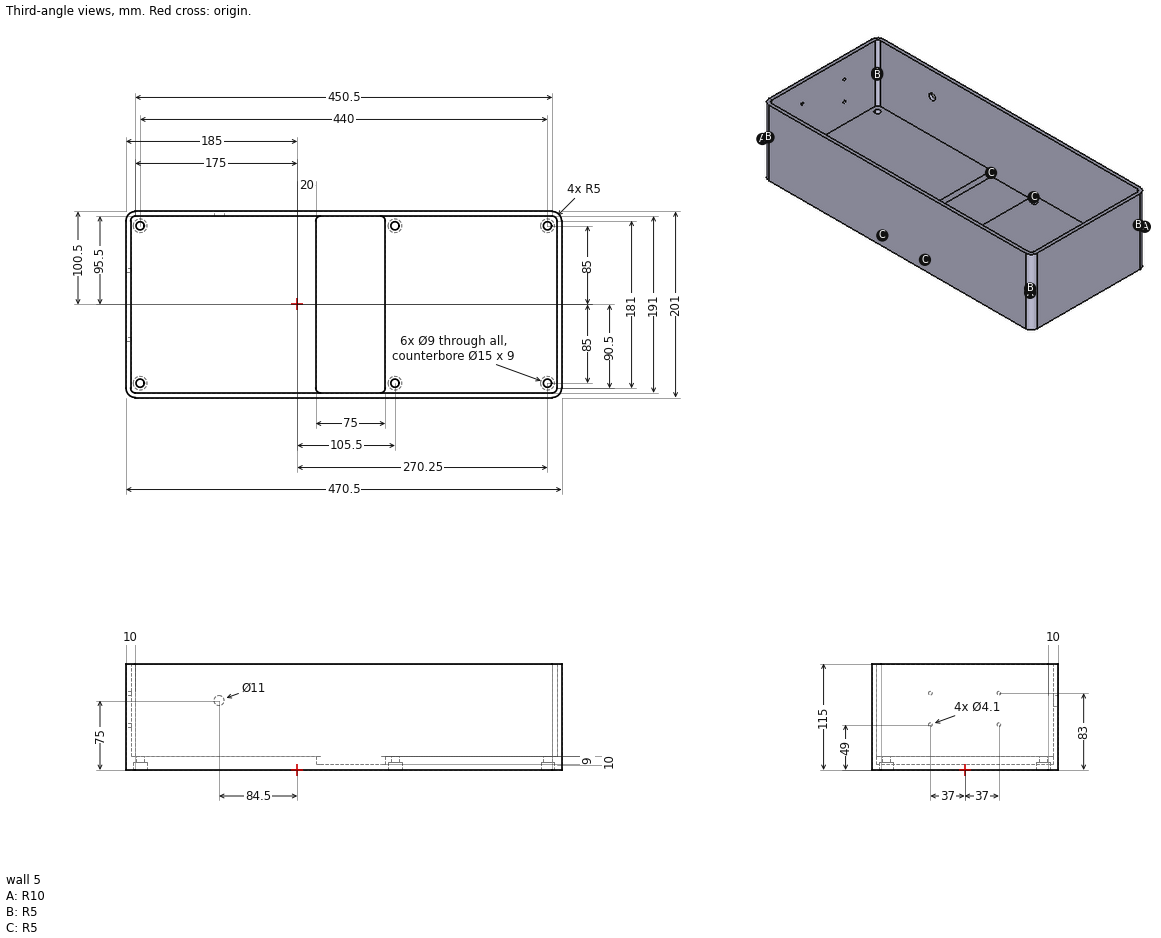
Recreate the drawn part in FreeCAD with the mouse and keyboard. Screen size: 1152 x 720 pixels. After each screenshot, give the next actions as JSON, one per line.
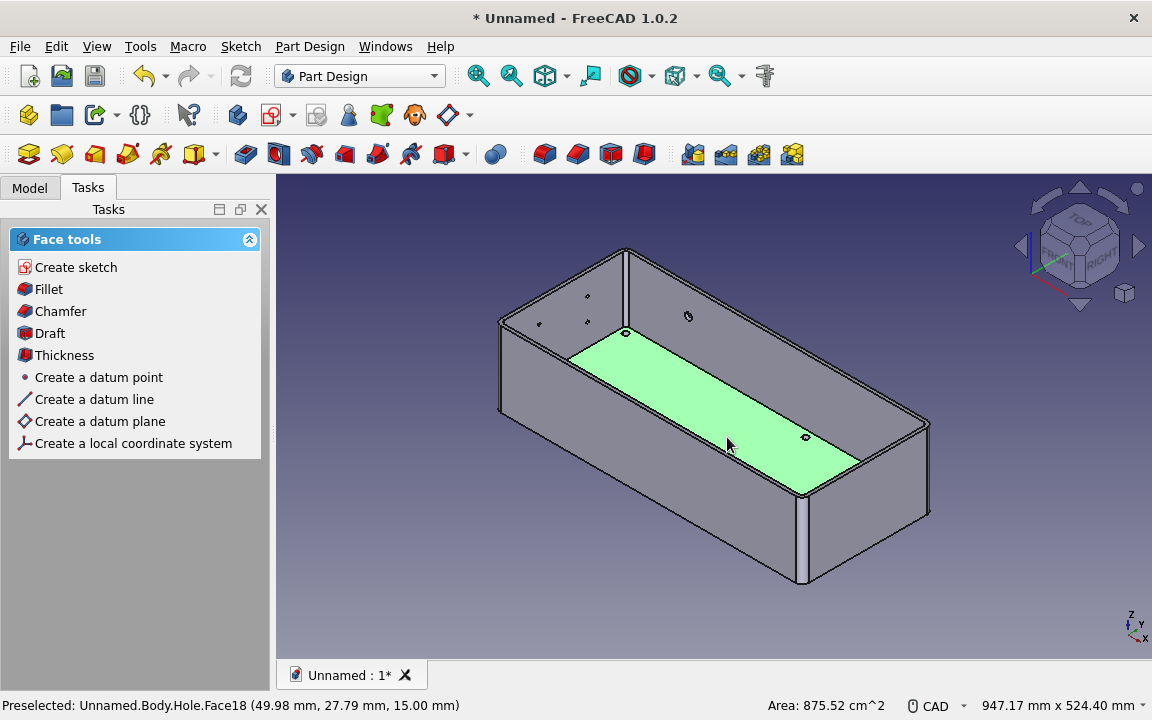
{"action": "left_click", "coordinate": [270, 116]}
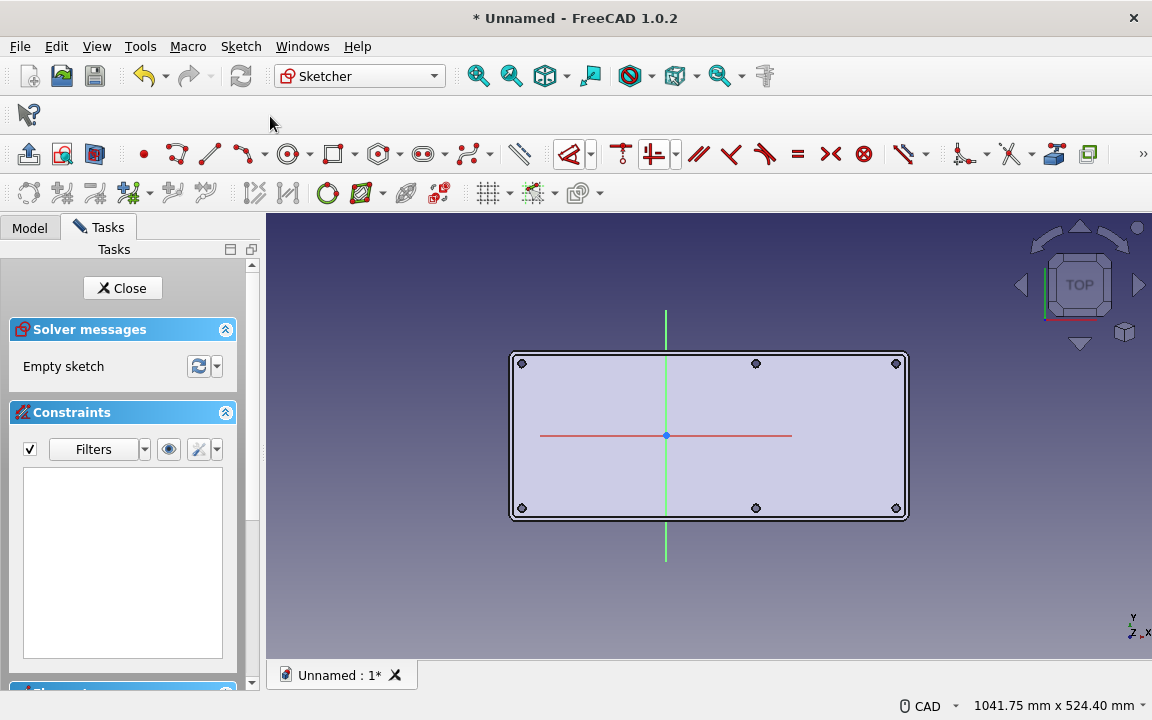
{"action": "scroll", "coordinate": [787, 436], "scroll_direction": "up", "scroll_amount": 3}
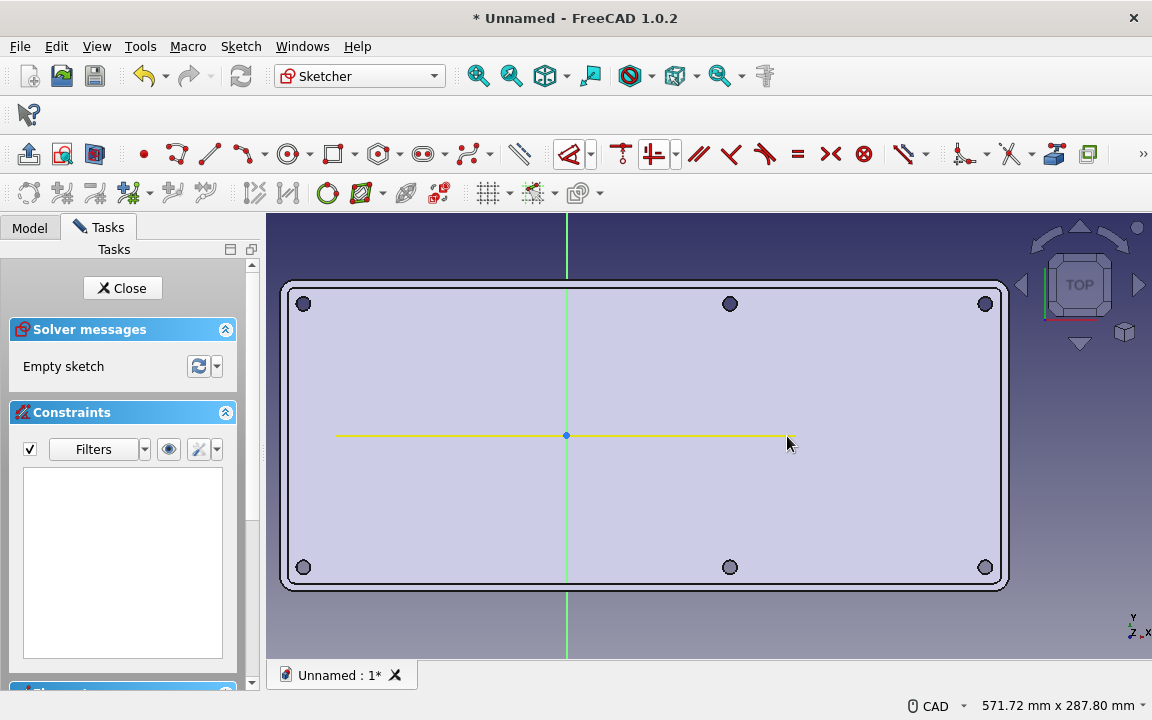
{"action": "left_click", "coordinate": [332, 154]}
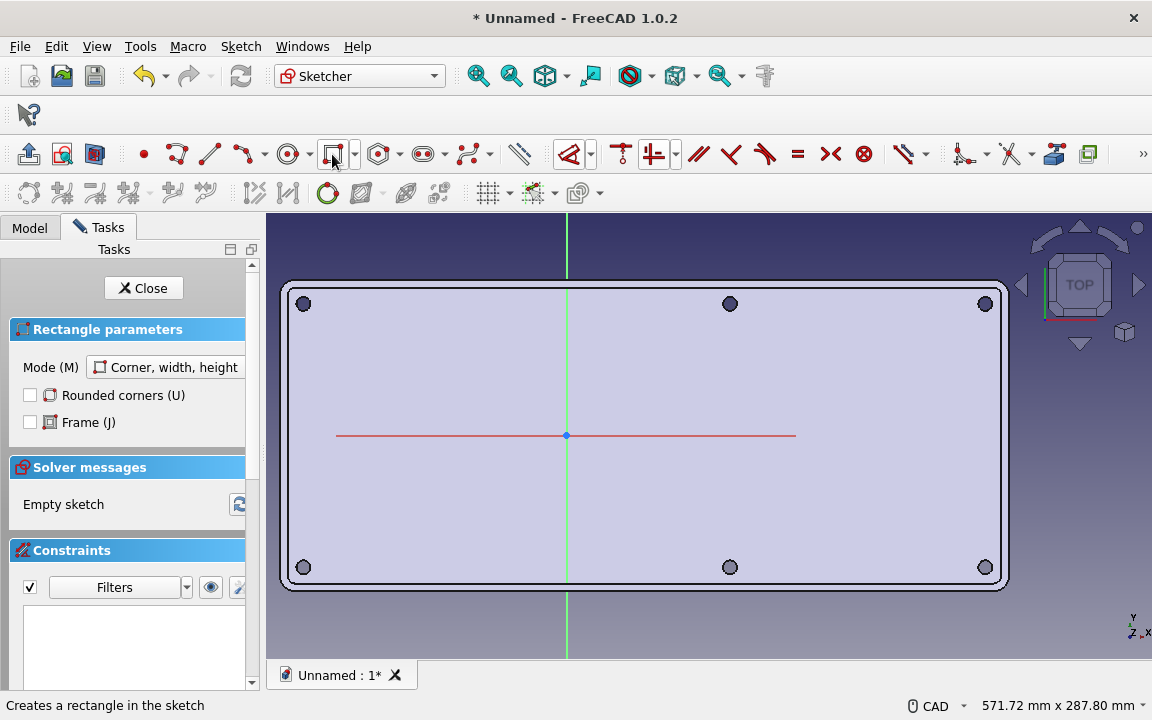
{"action": "left_click", "coordinate": [598, 288]}
{"action": "mouse_move", "coordinate": [714, 584]}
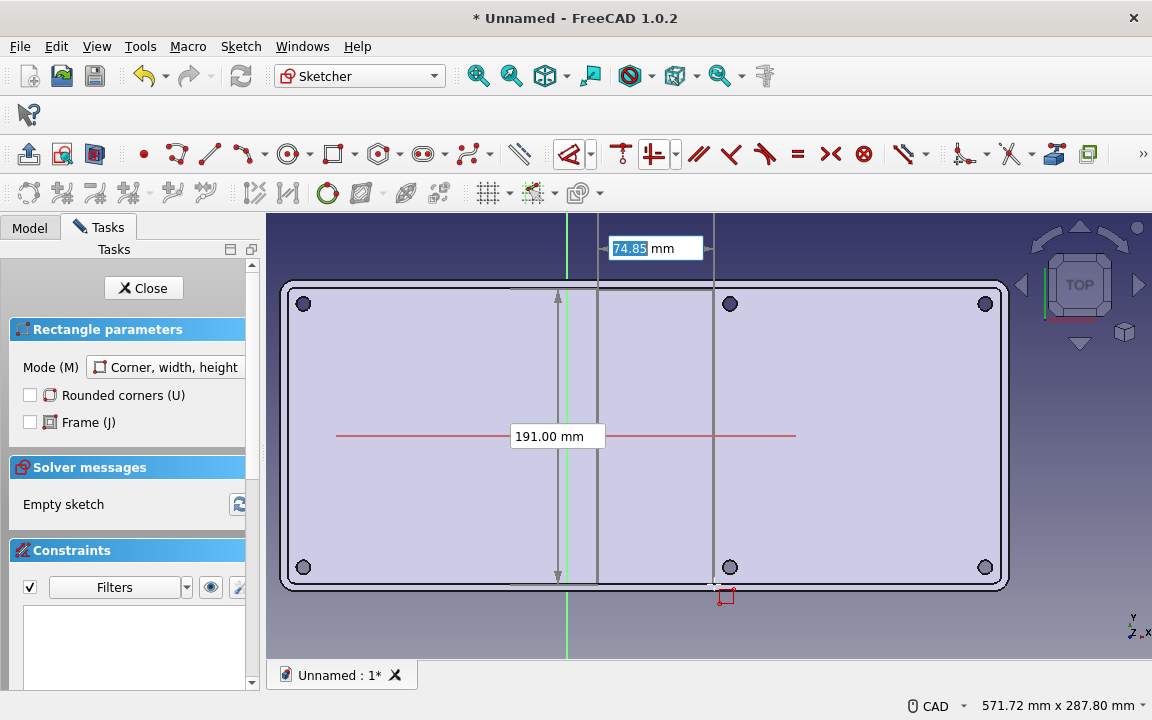
{"action": "type", "text": "75"}
{"action": "key", "text": "Tab"}
{"action": "type", "text": "191"}
{"action": "key", "text": "Return"}
{"action": "key", "text": "Escape"}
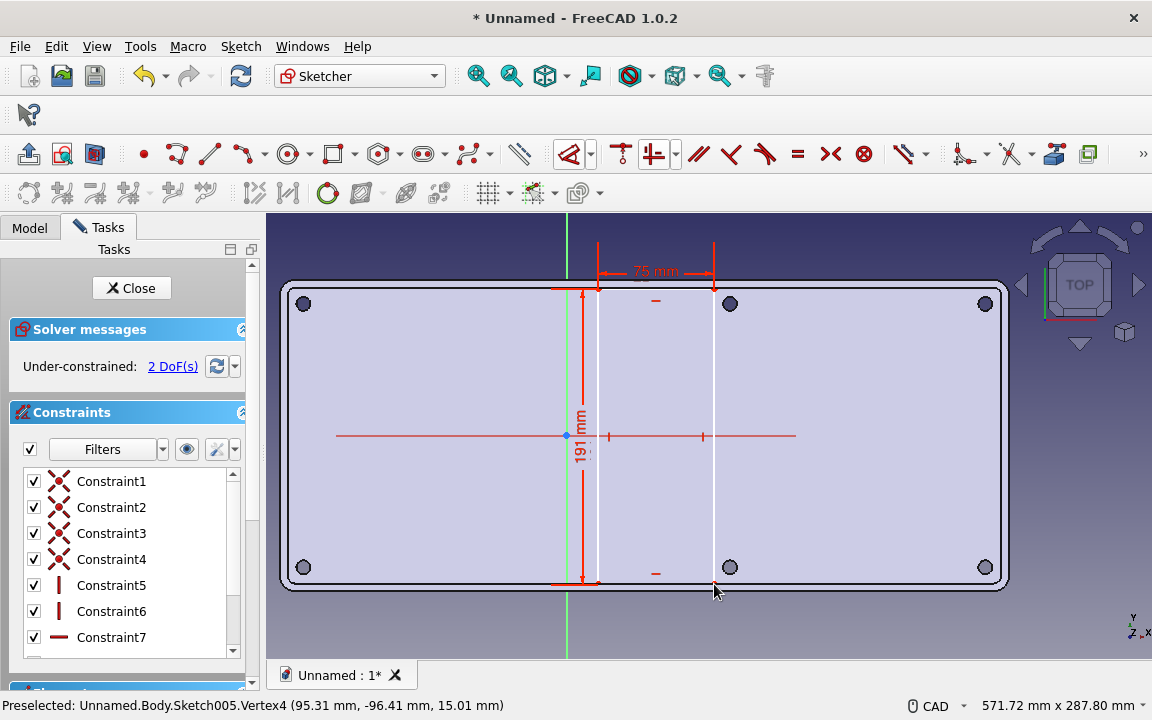
{"action": "key", "text": "d"}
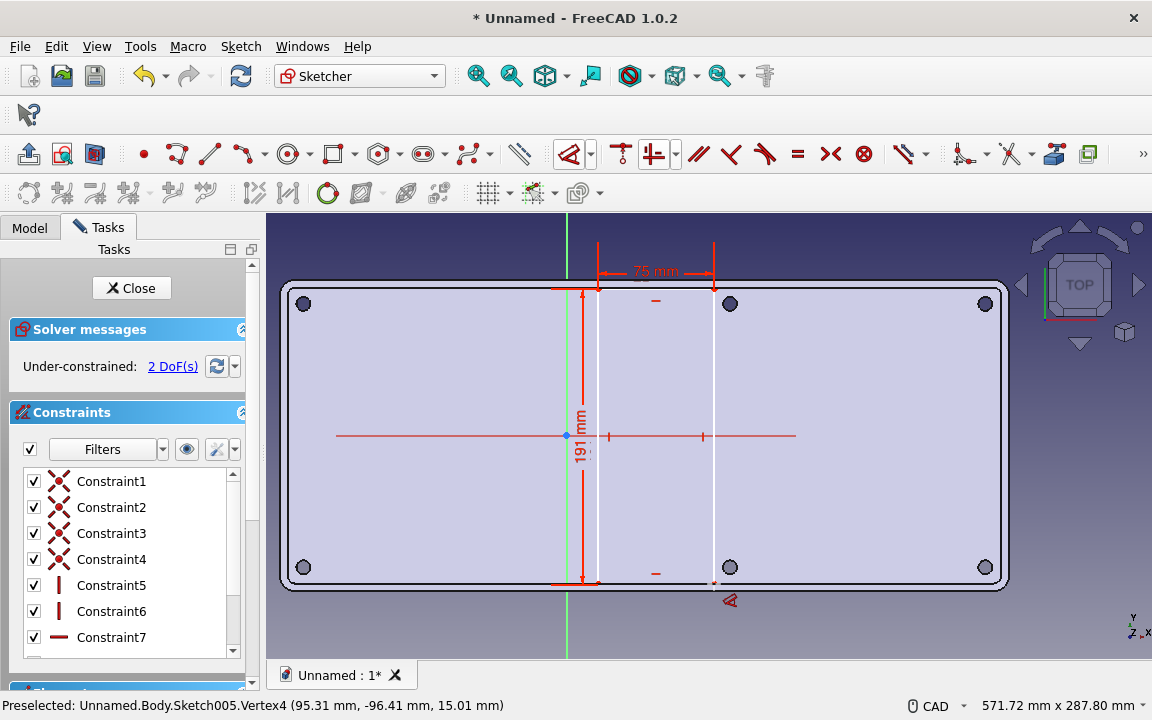
{"action": "scroll", "coordinate": [598, 289], "scroll_direction": "up", "scroll_amount": 2}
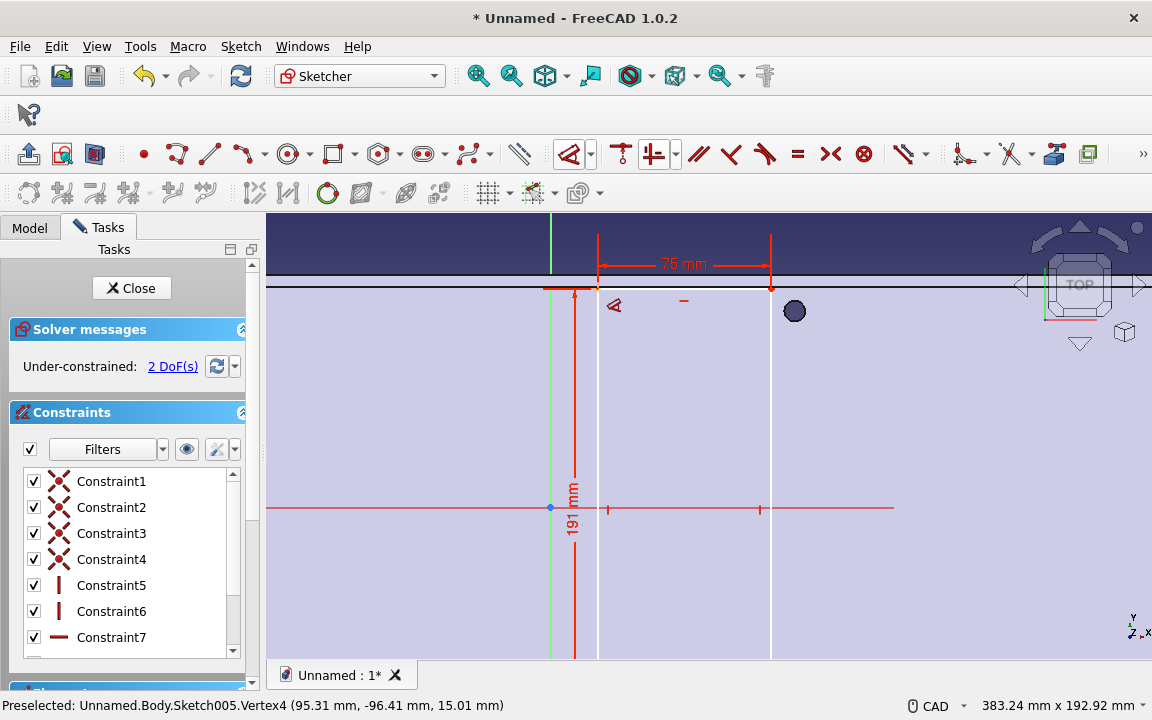
{"action": "left_click", "coordinate": [598, 289]}
{"action": "left_click", "coordinate": [574, 255]}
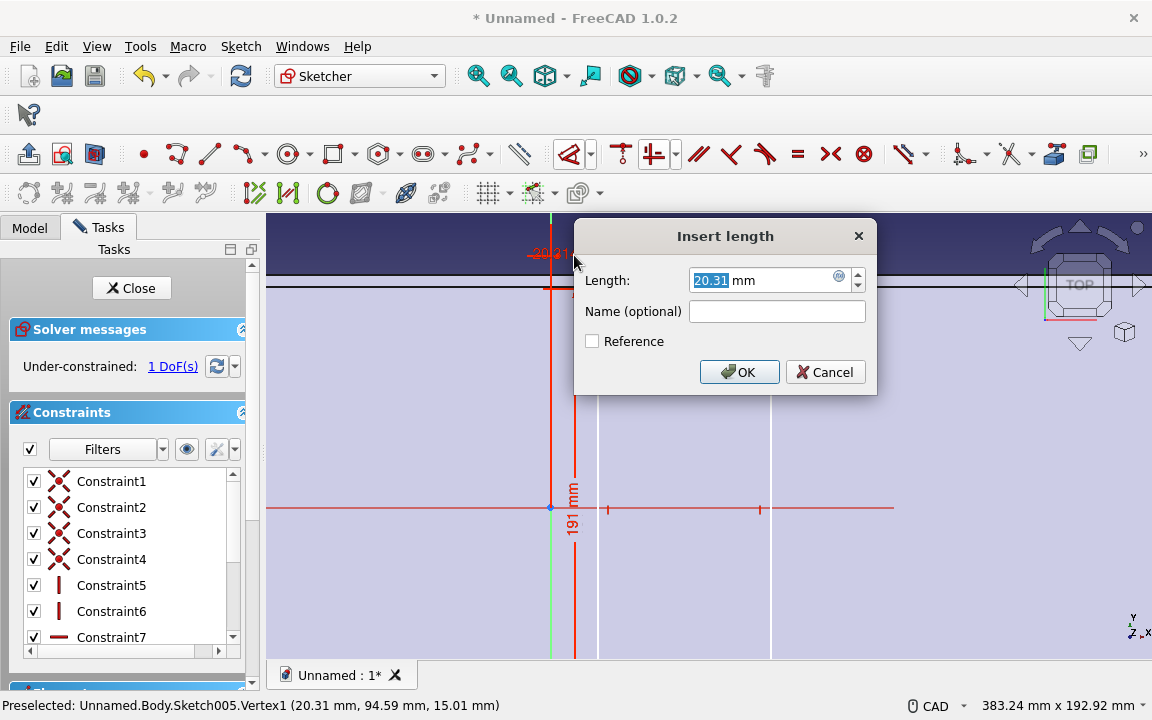
{"action": "type", "text": "20"}
{"action": "key", "text": "Return"}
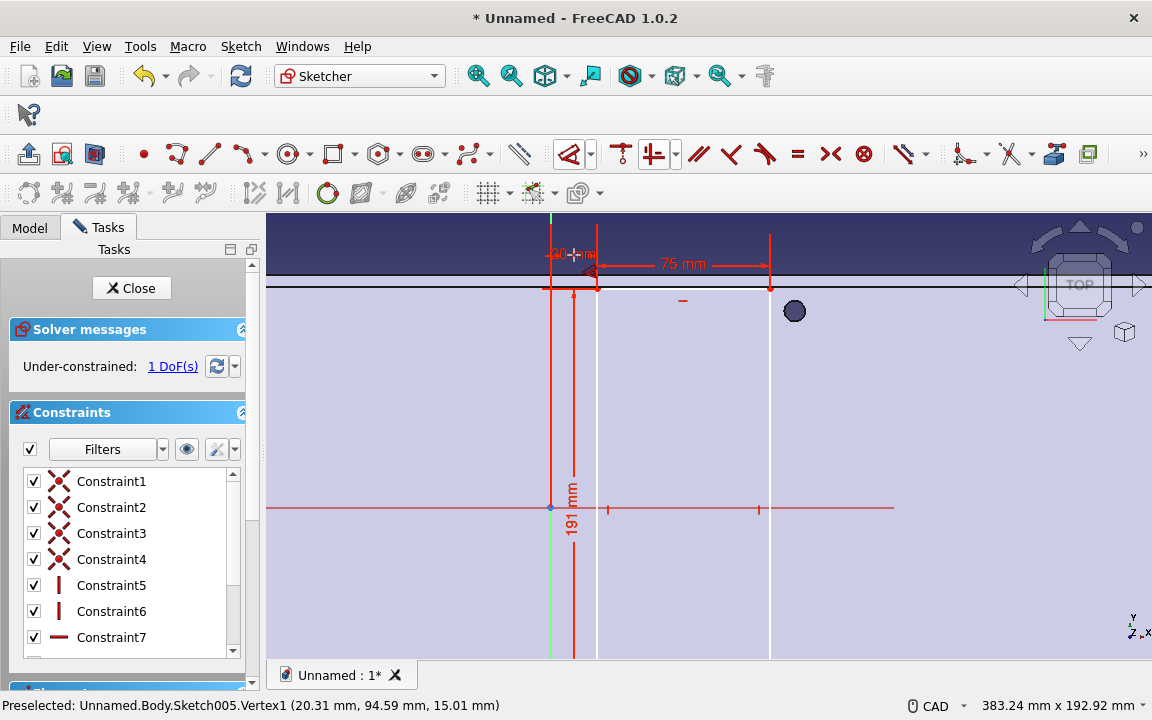
{"action": "left_click", "coordinate": [597, 289]}
{"action": "left_click", "coordinate": [517, 398]}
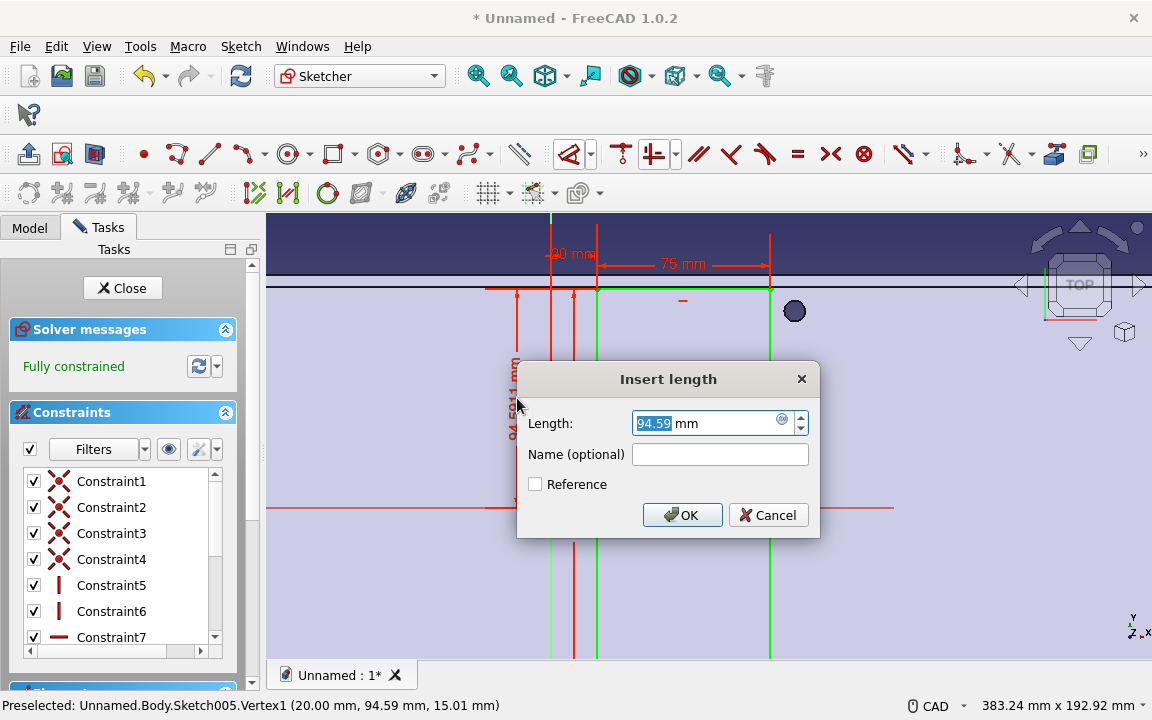
{"action": "type", "text": "95.5"}
{"action": "key", "text": "Return"}
{"action": "key", "text": "Escape"}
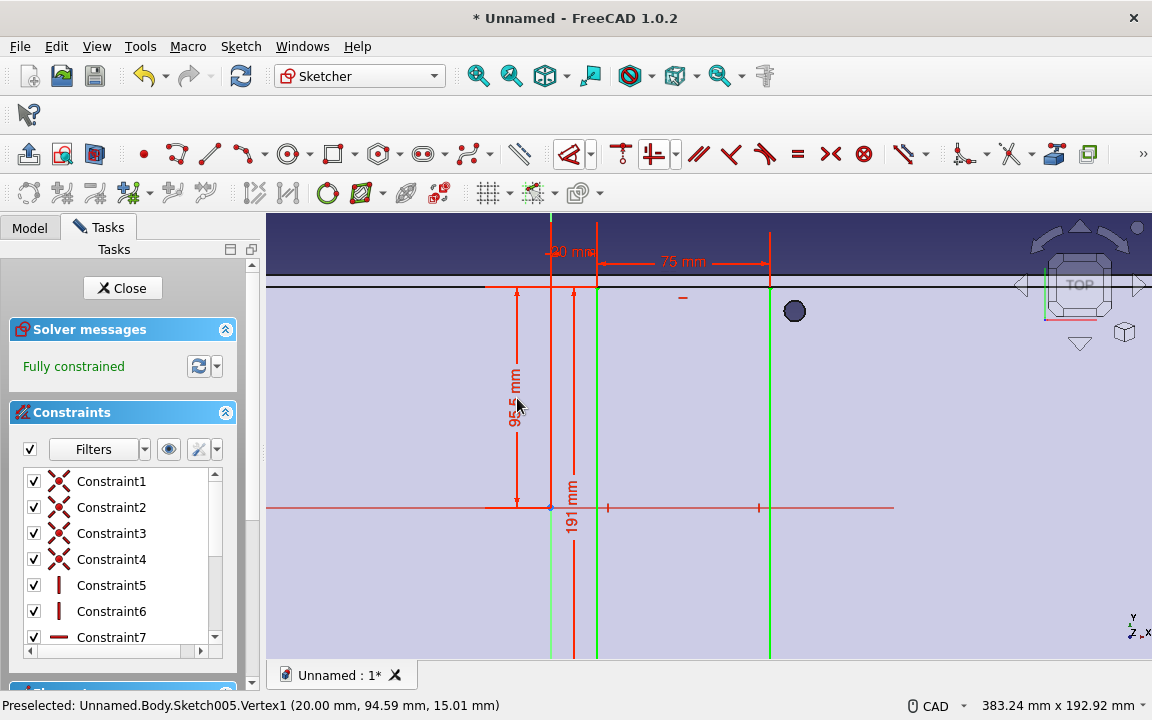
{"action": "left_click", "coordinate": [123, 288]}